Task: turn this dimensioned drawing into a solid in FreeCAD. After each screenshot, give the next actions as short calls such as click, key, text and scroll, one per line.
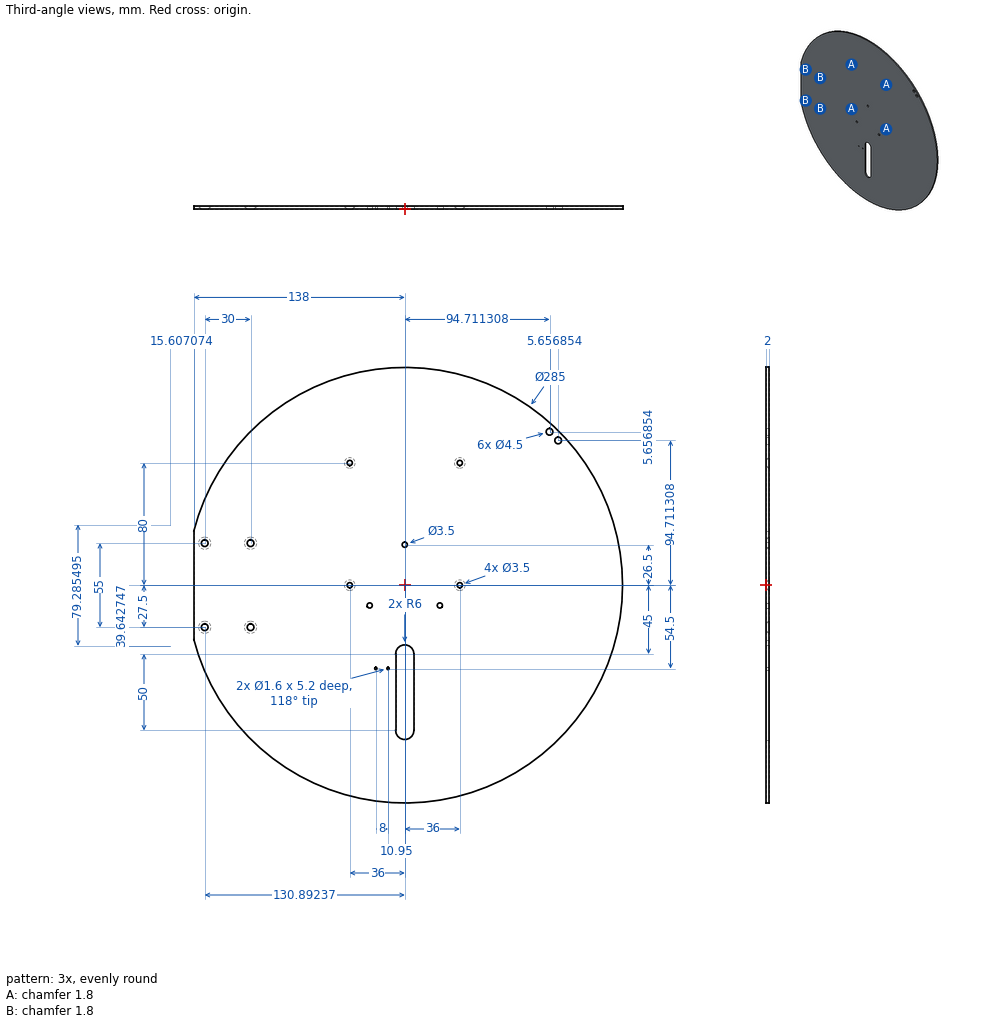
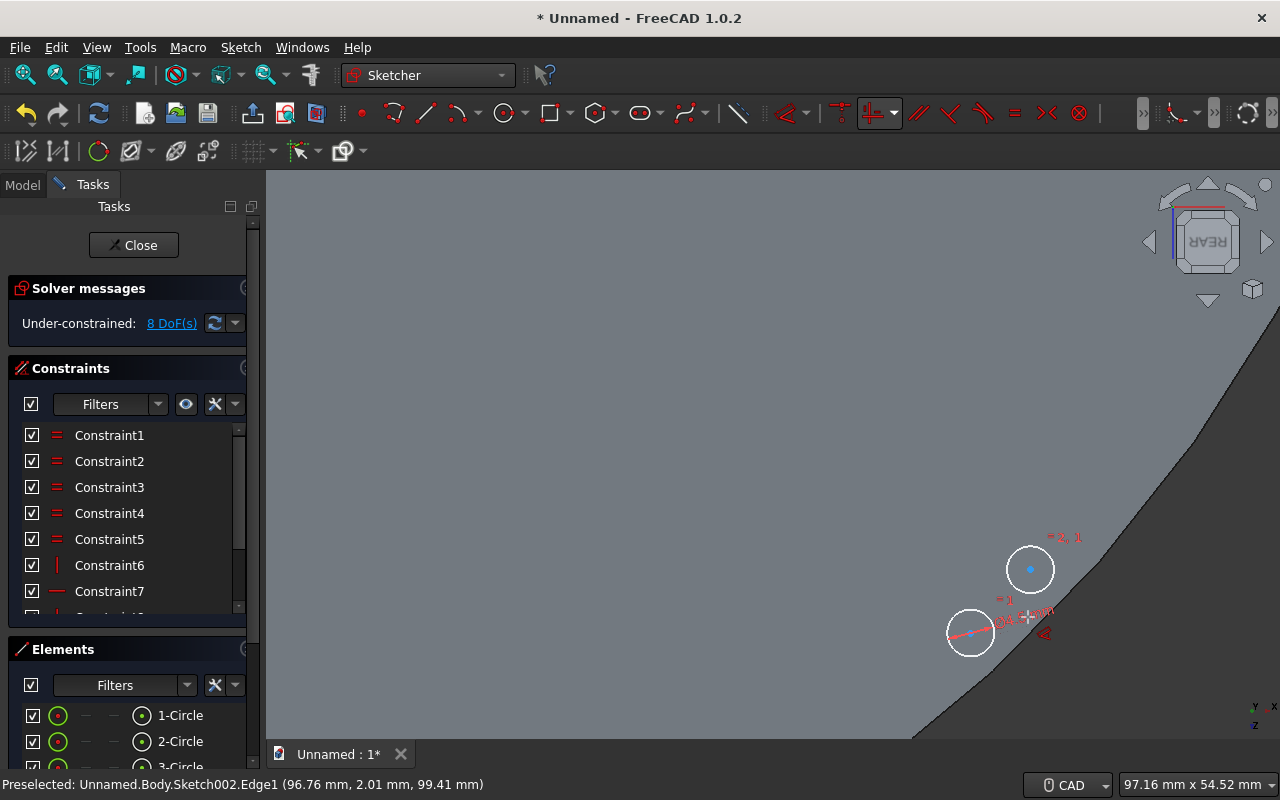
scroll(993, 616, down, 7)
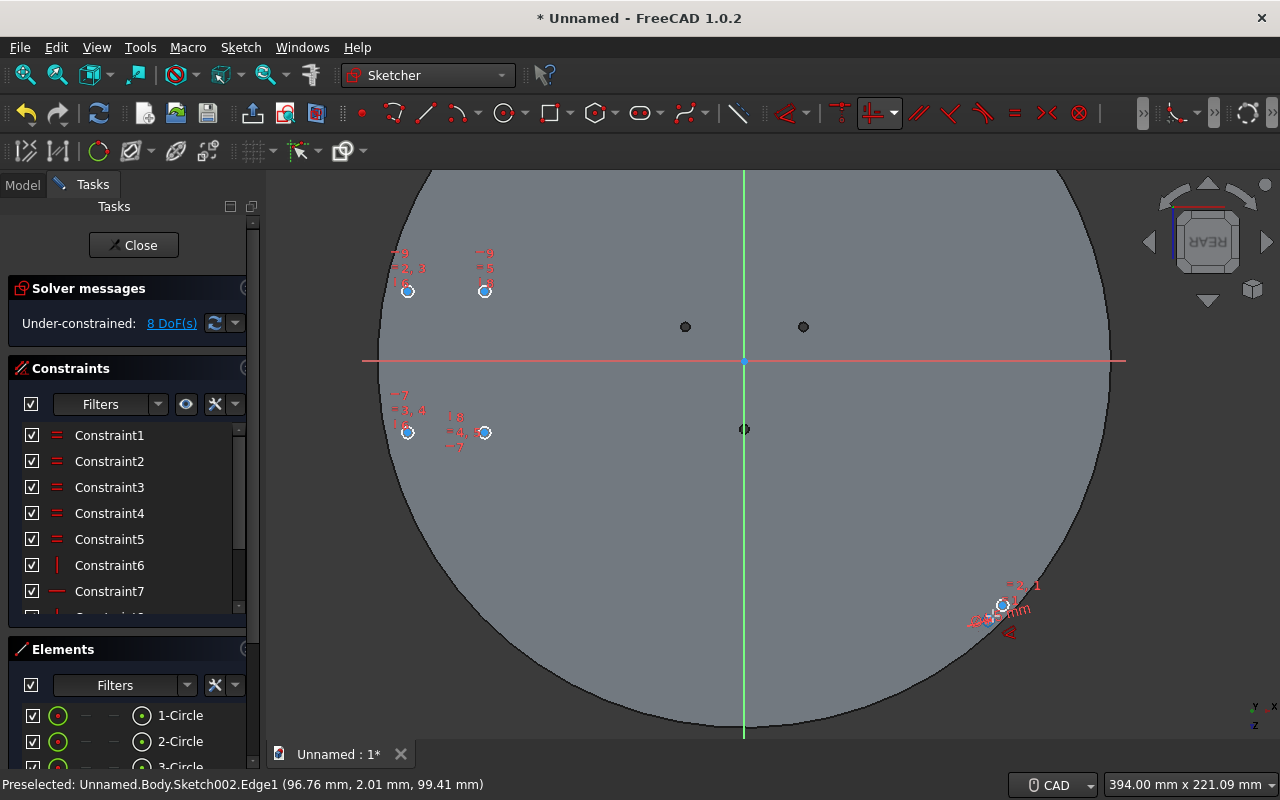
click(408, 292)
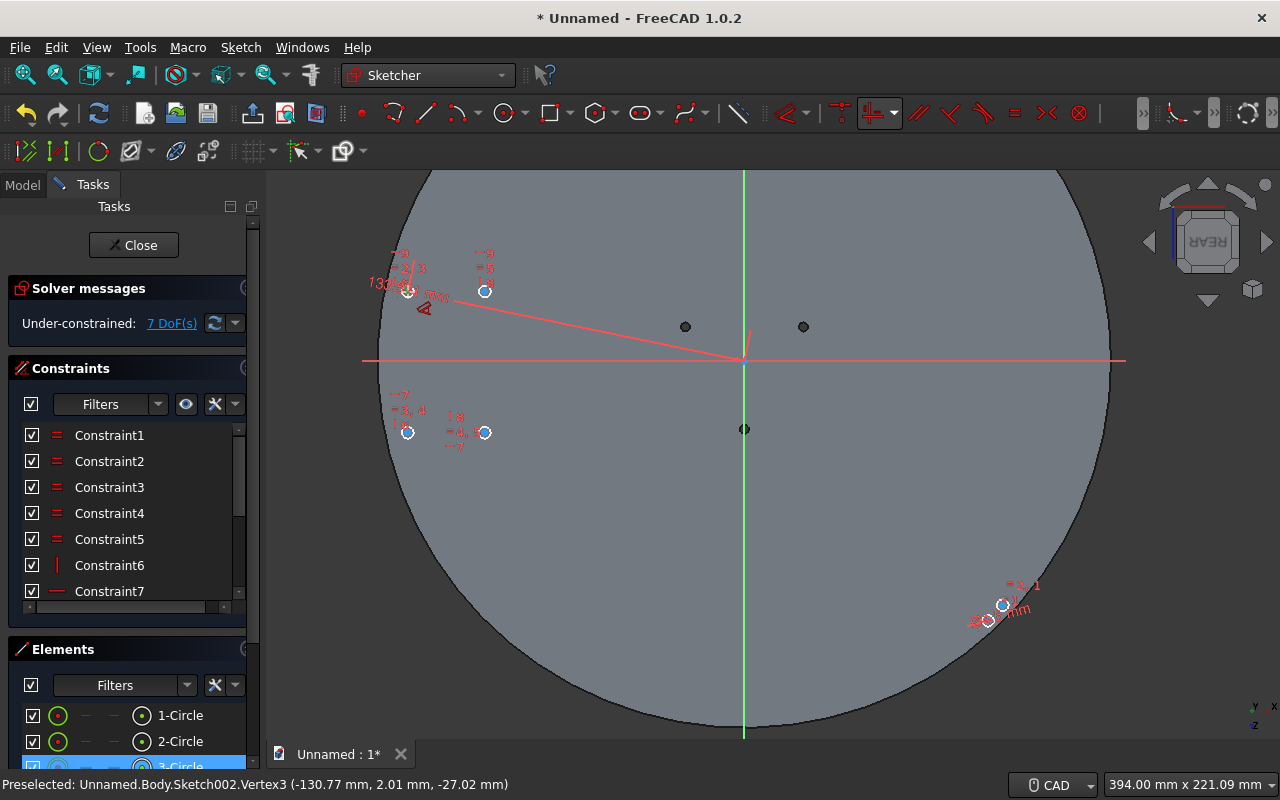
click(408, 433)
click(374, 330)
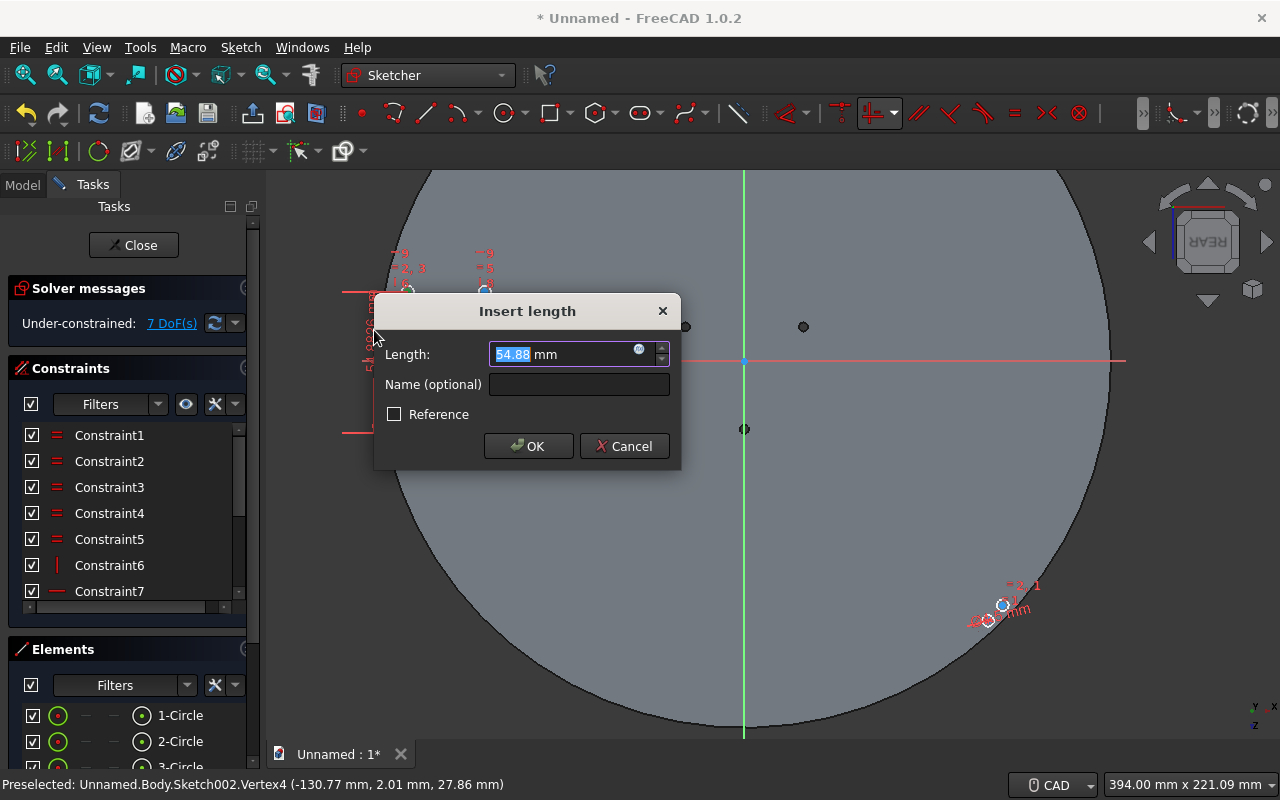
text(55)
key(Return)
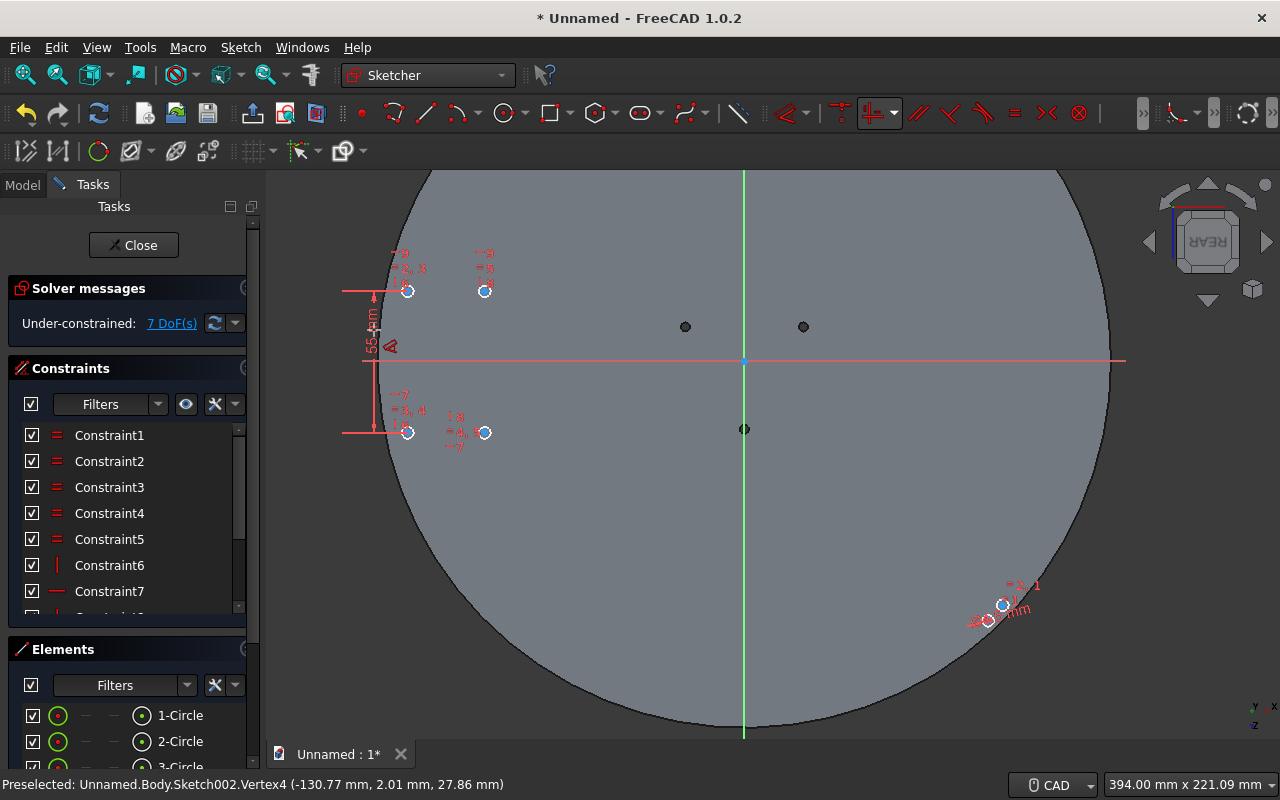
click(408, 433)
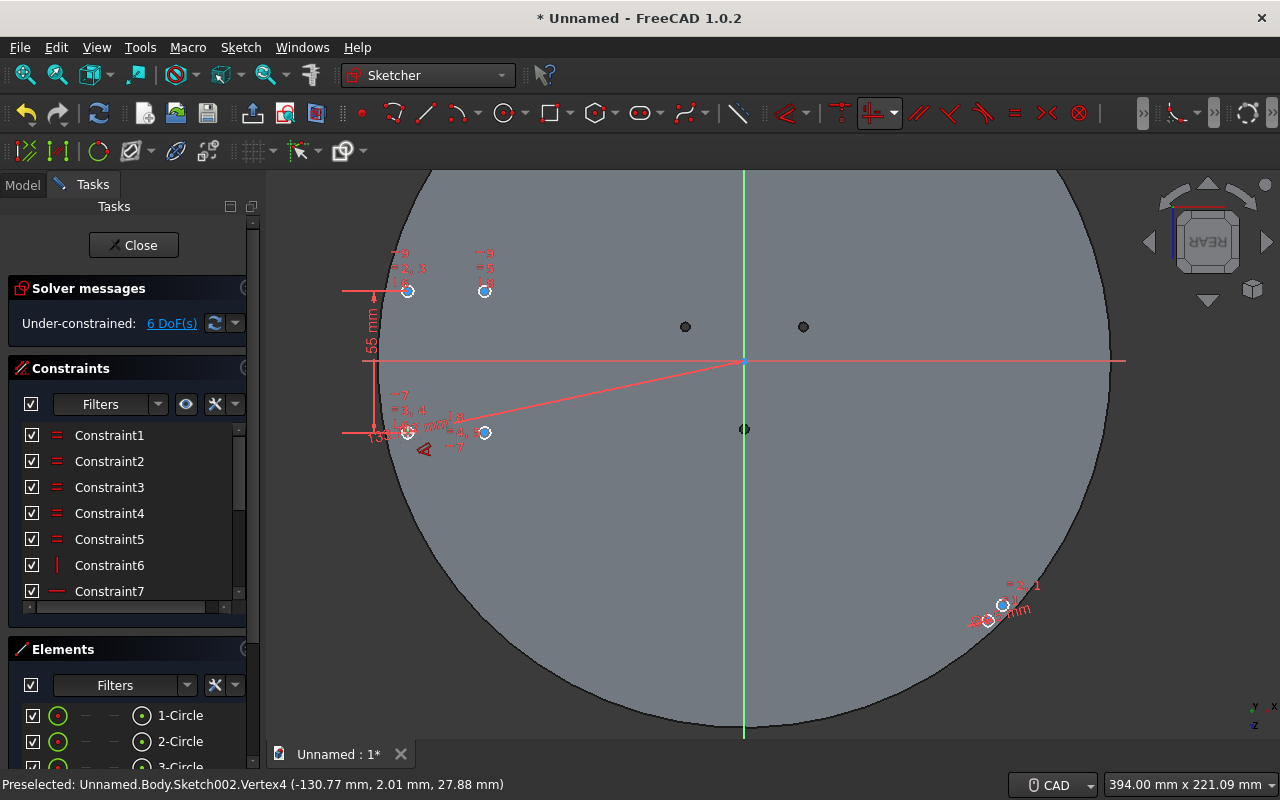
click(485, 433)
click(446, 399)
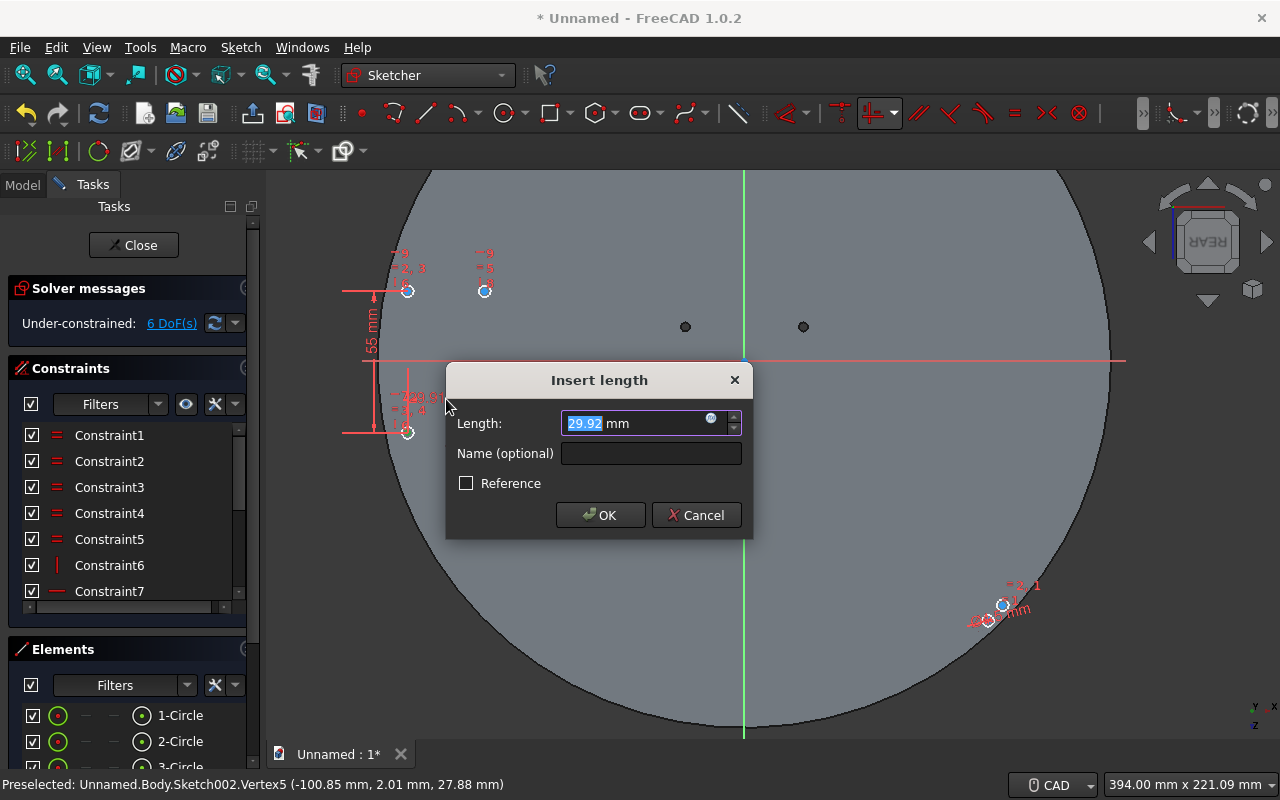
text(30)
key(Return)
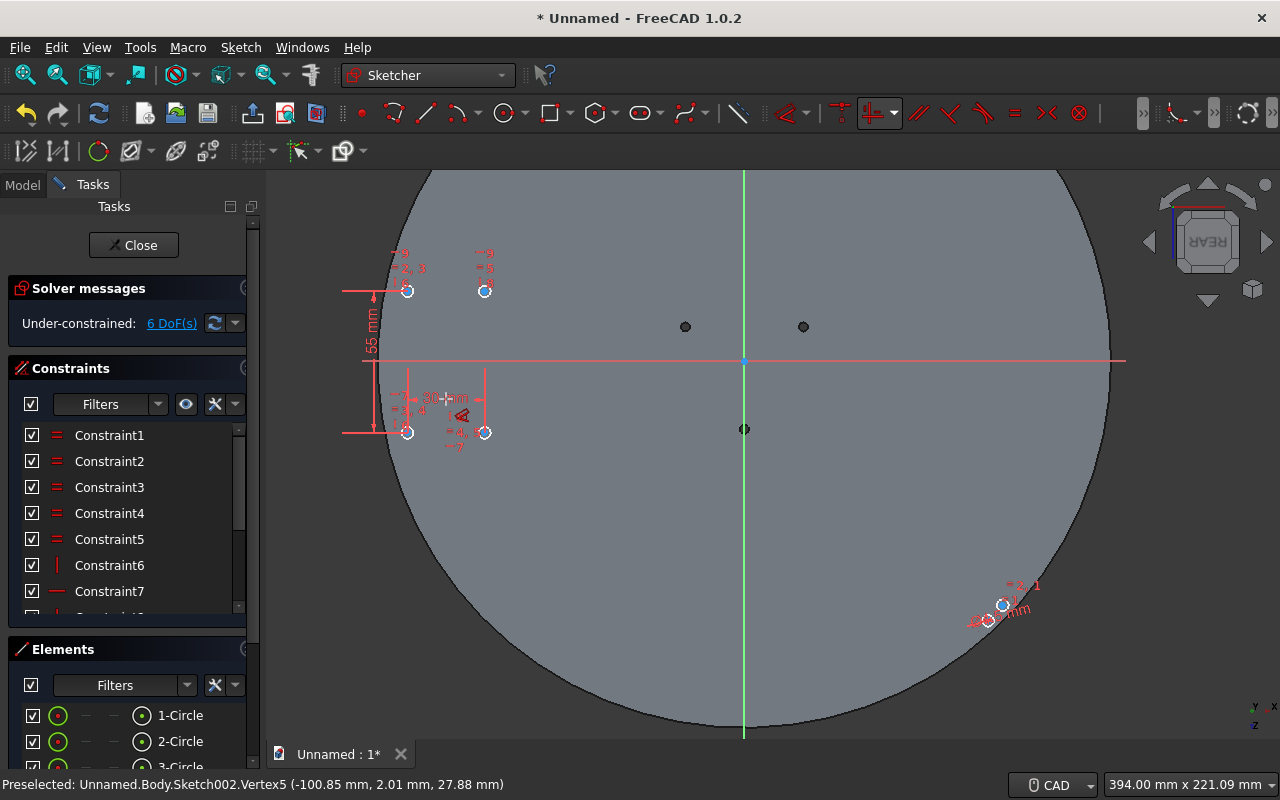
click(408, 291)
click(374, 302)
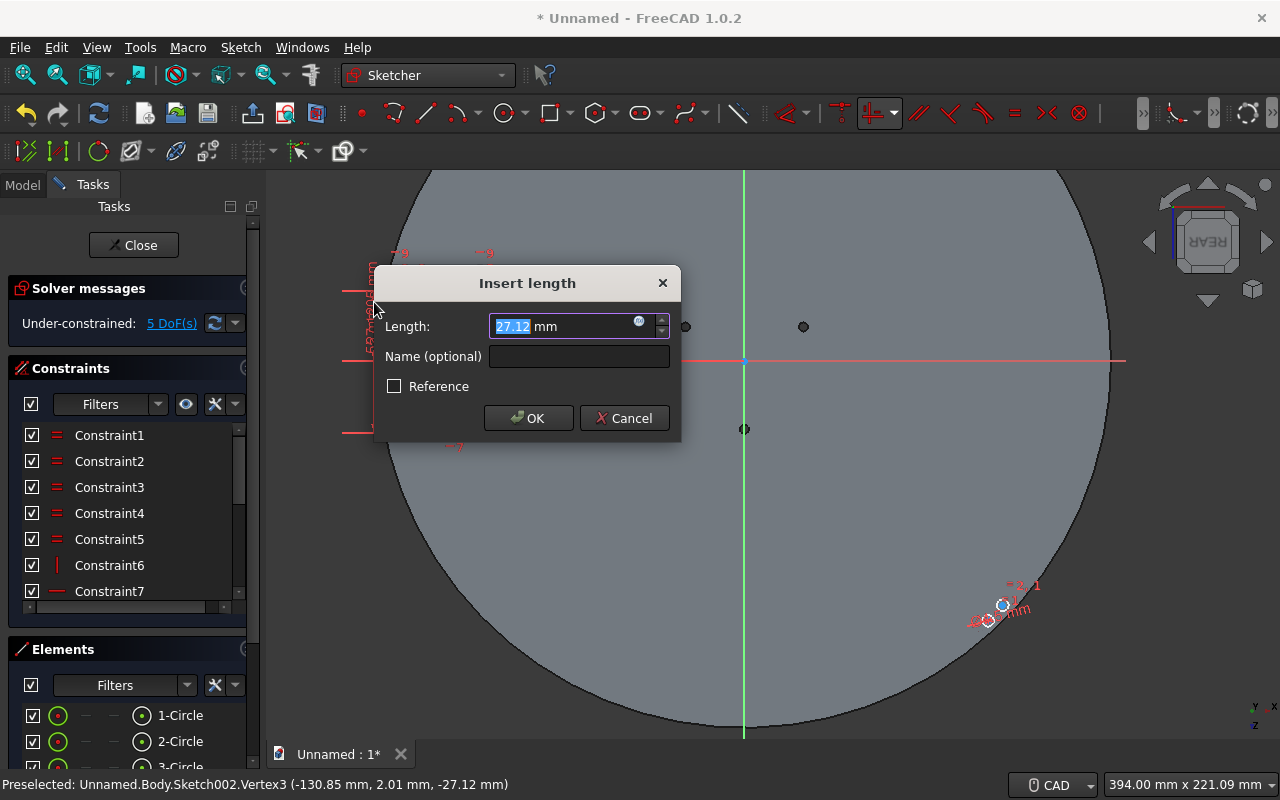
text(27.5)
key(Return)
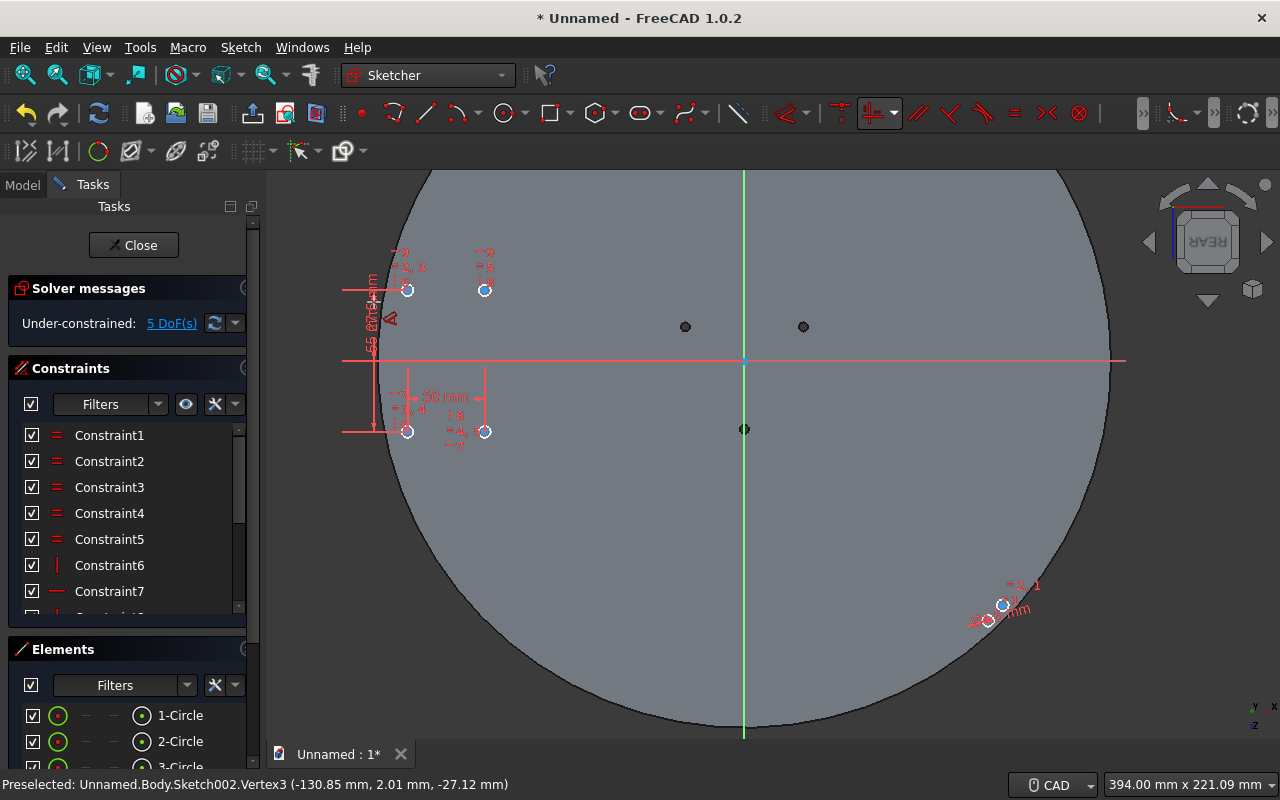
click(988, 621)
click(866, 655)